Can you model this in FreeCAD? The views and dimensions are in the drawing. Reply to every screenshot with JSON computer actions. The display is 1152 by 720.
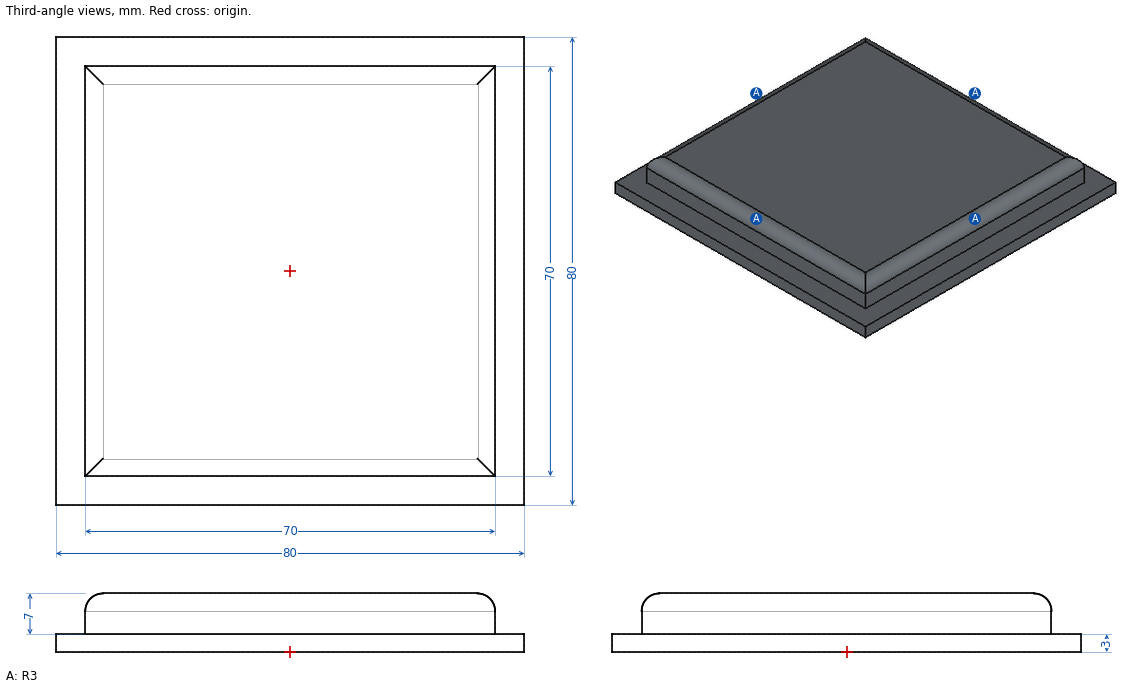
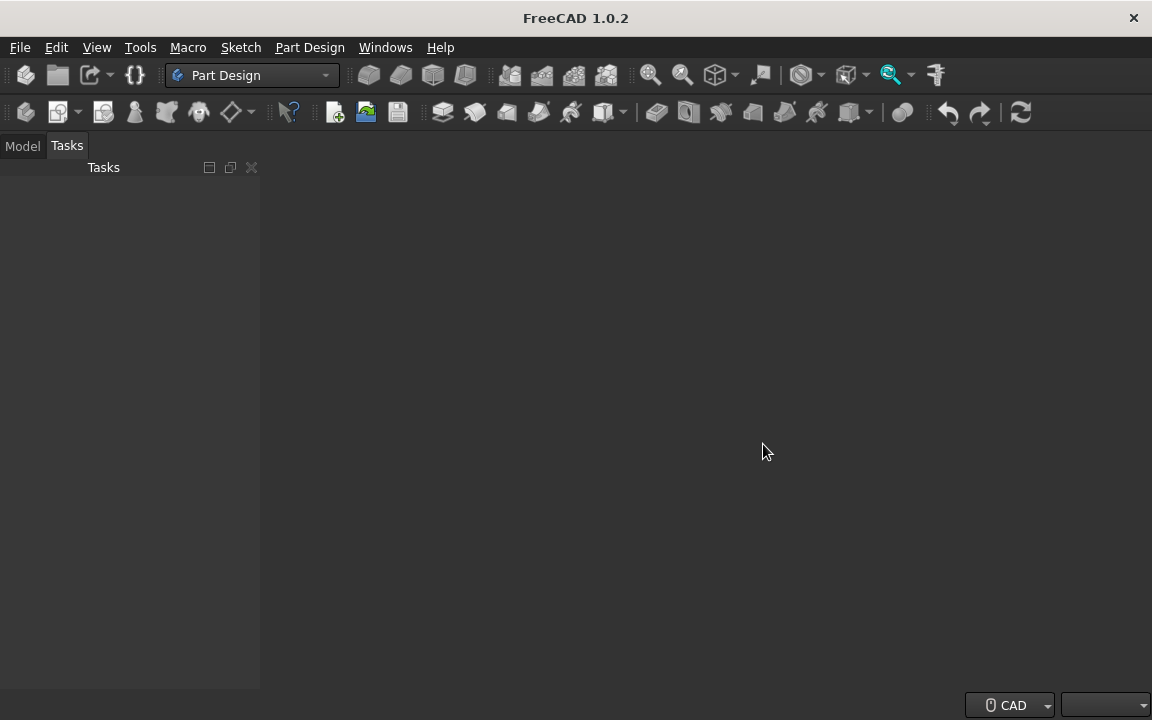
{"action": "left_click", "coordinate": [334, 112]}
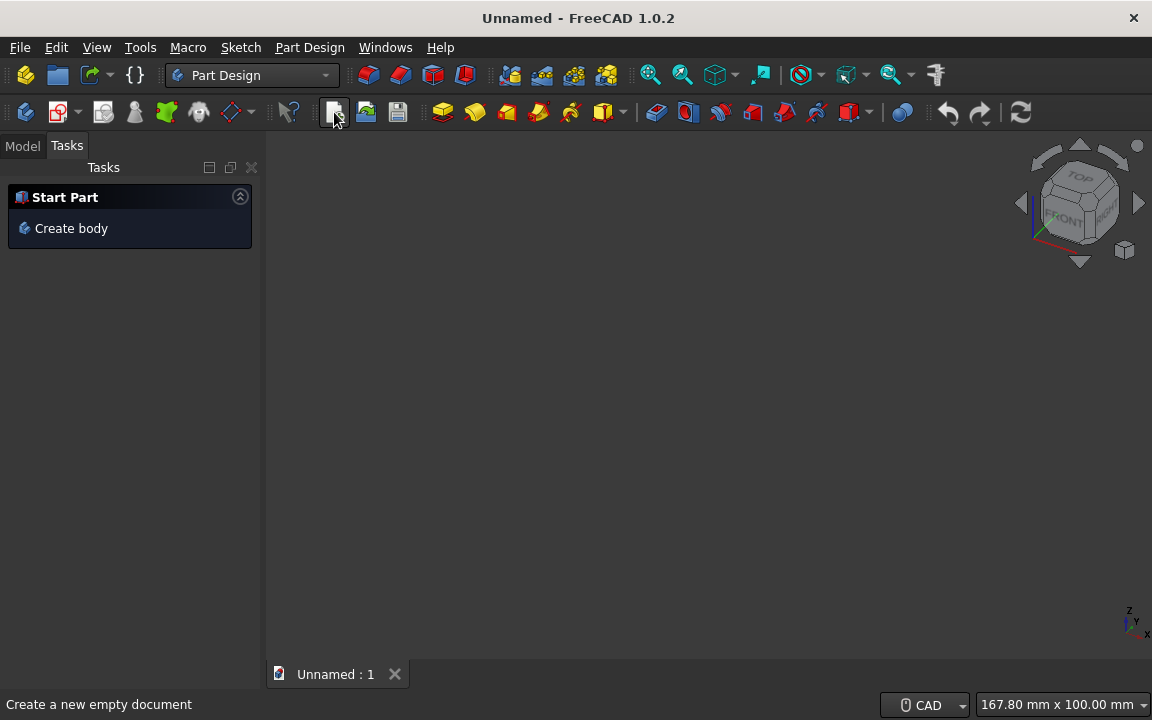
{"action": "left_click", "coordinate": [58, 112]}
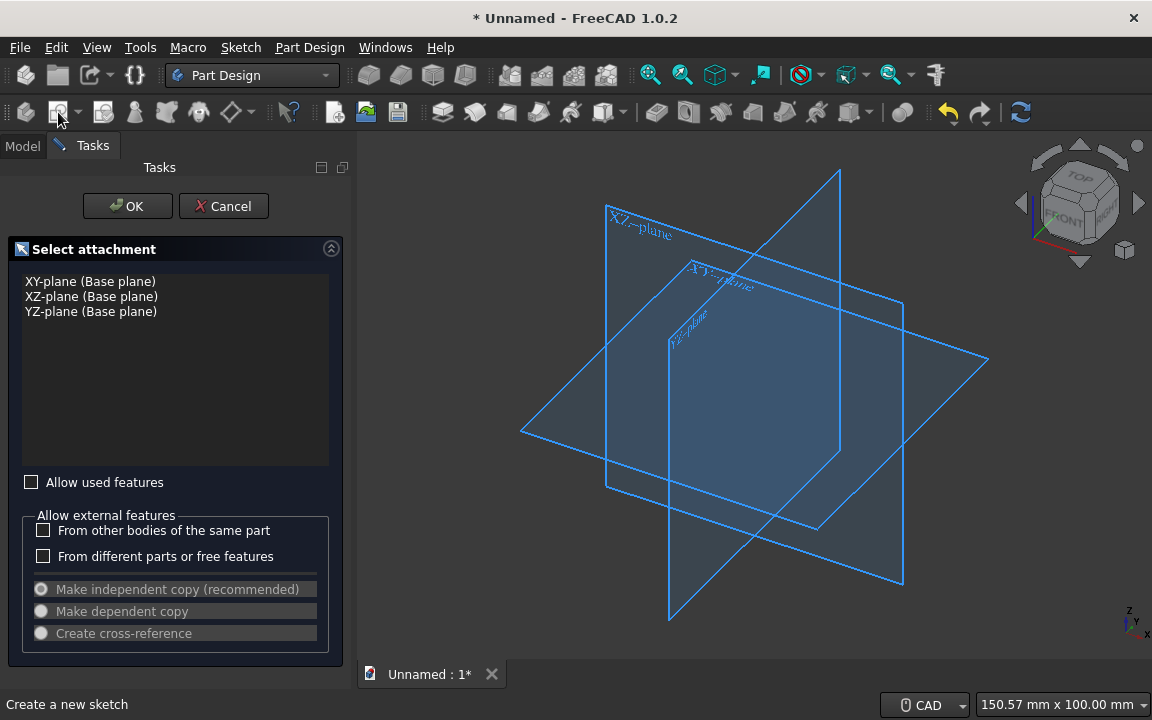
{"action": "left_click", "coordinate": [82, 282]}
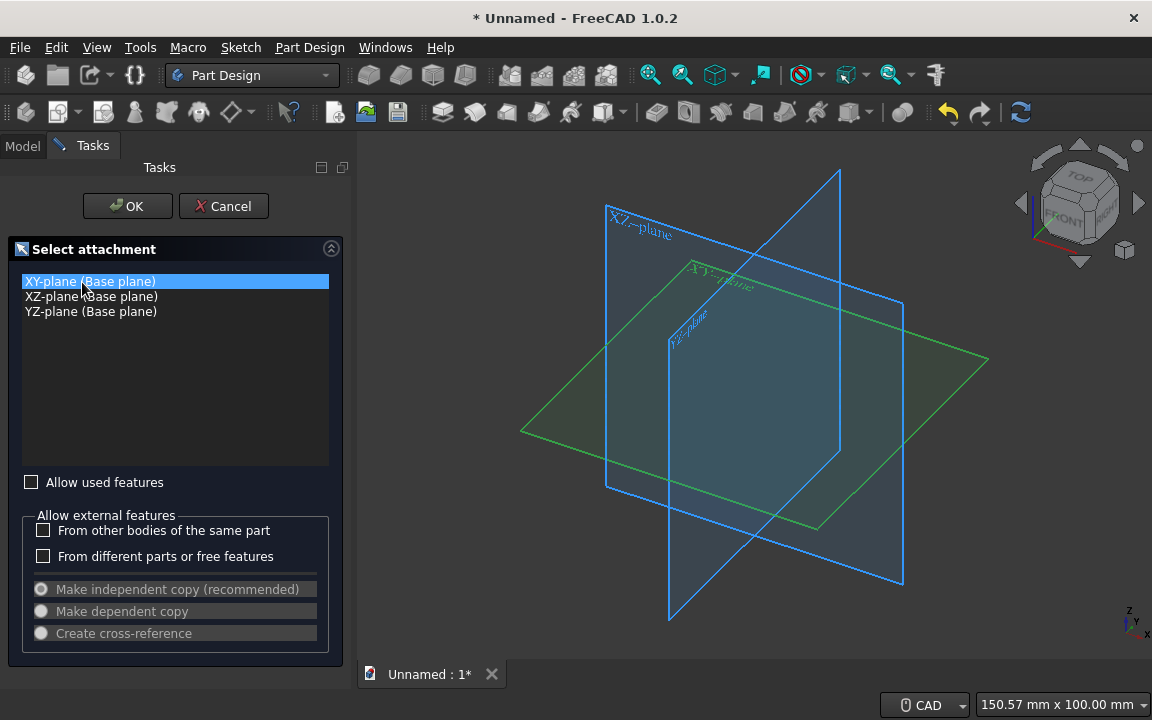
{"action": "left_click", "coordinate": [128, 206]}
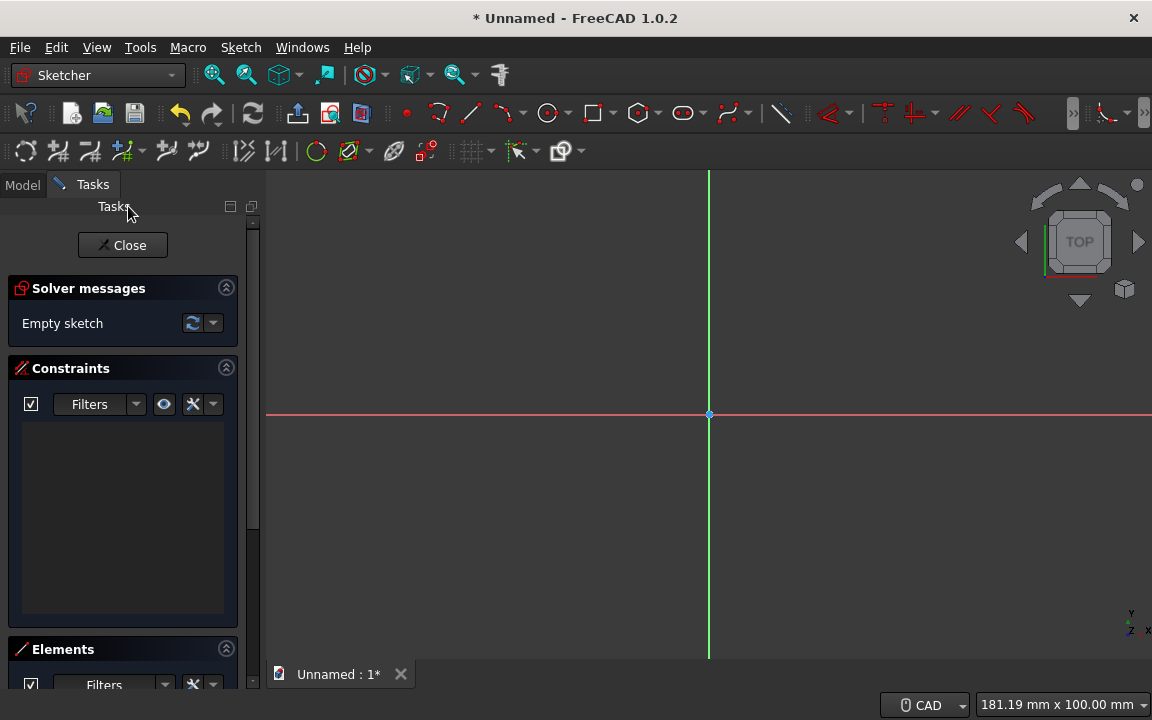
{"action": "scroll", "coordinate": [331, 415], "scroll_direction": "down", "scroll_amount": 1}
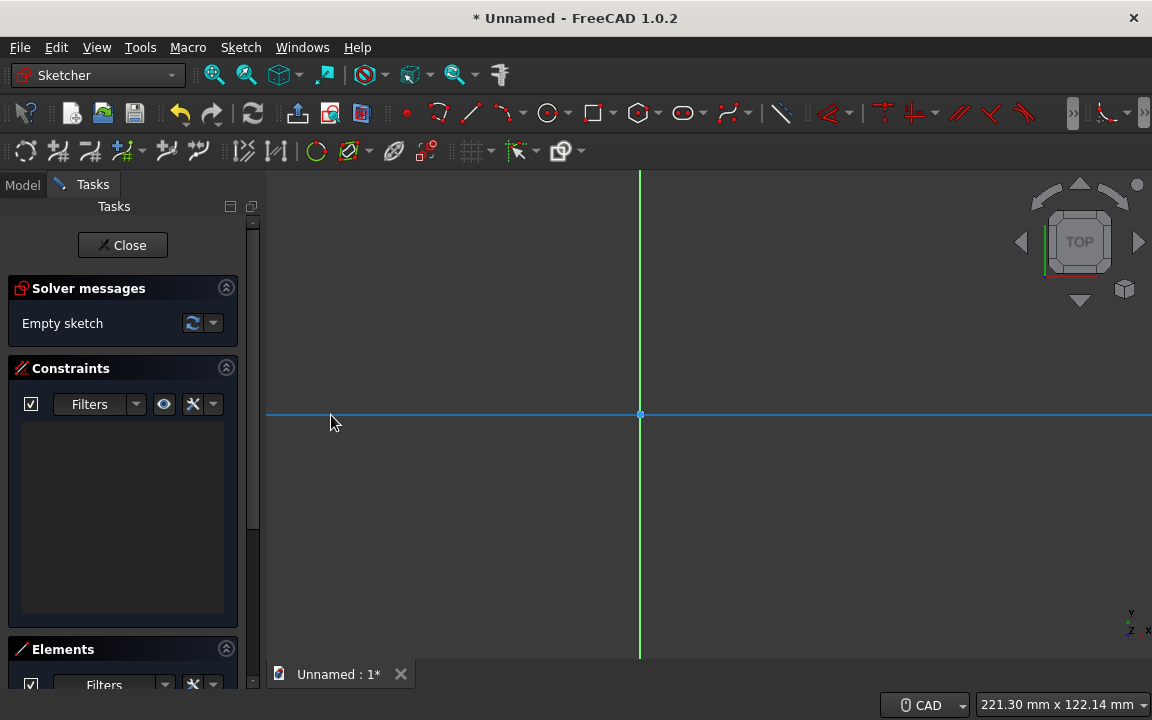
{"action": "left_click", "coordinate": [616, 114]}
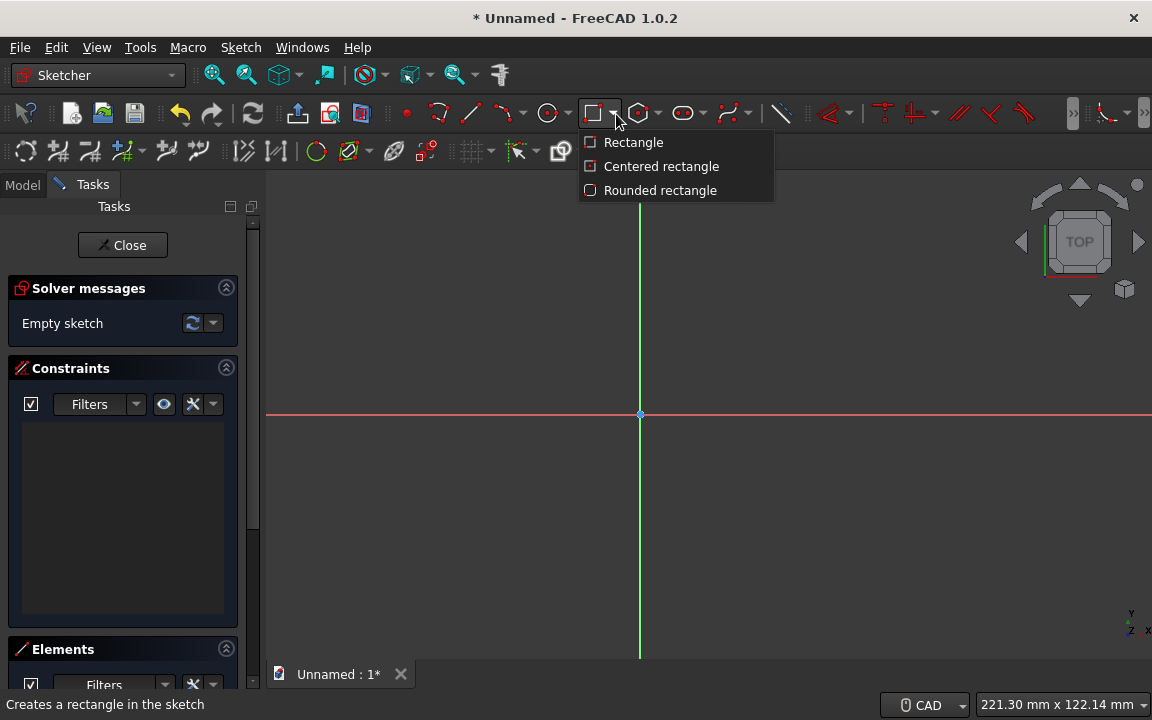
{"action": "left_click", "coordinate": [676, 166]}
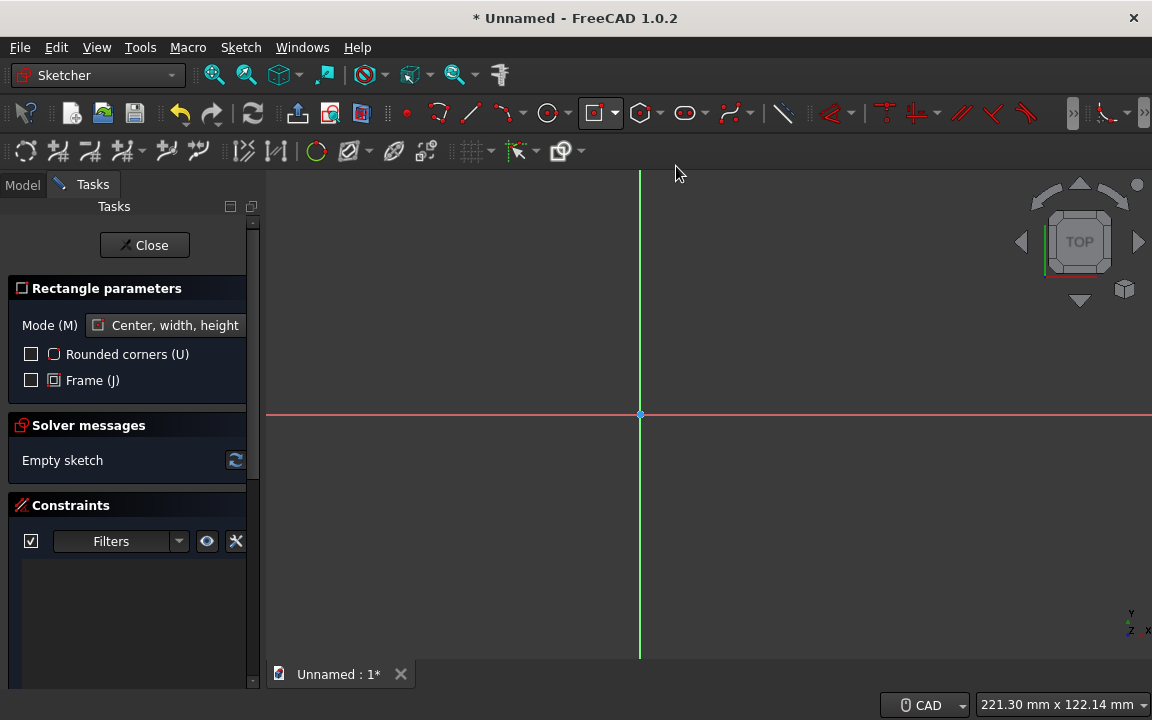
{"action": "left_click", "coordinate": [640, 415]}
{"action": "left_click", "coordinate": [801, 255]}
{"action": "key", "text": "Escape"}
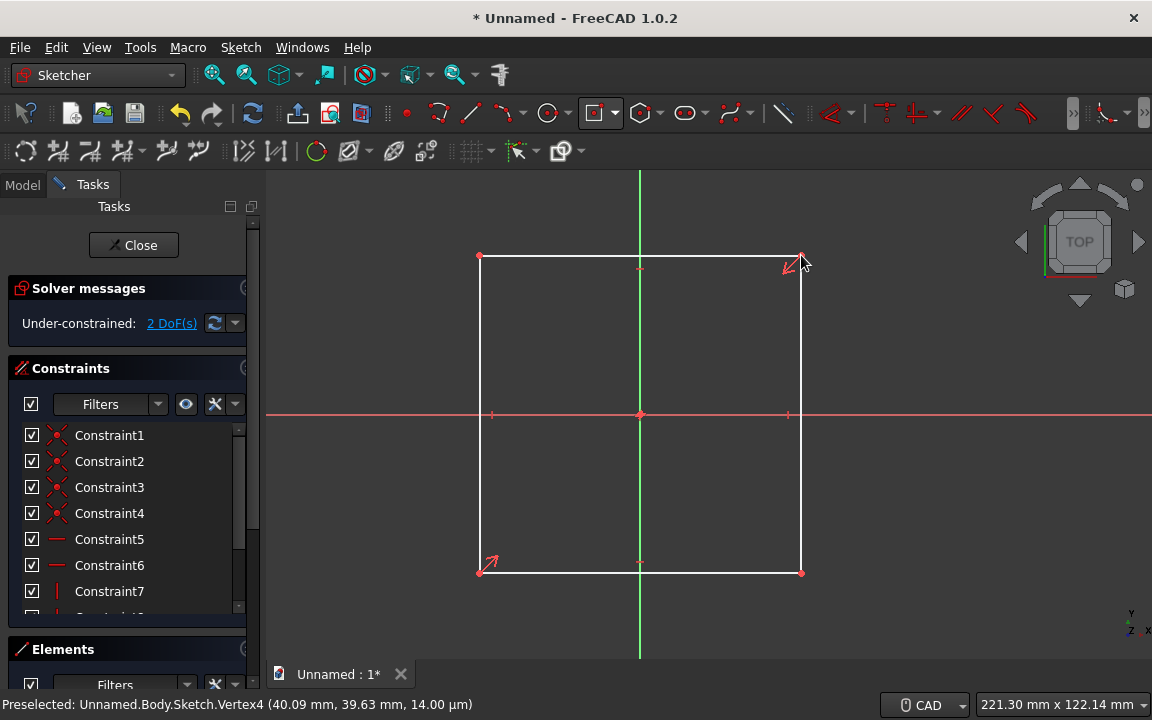
{"action": "left_click", "coordinate": [830, 114]}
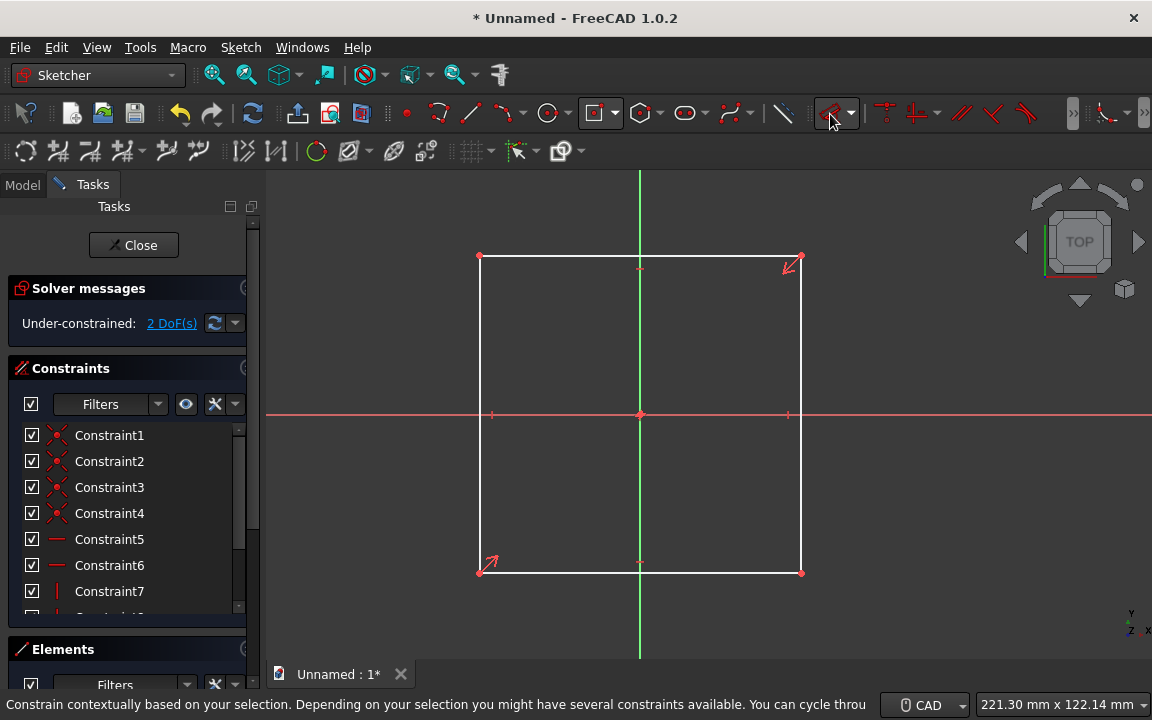
{"action": "left_click", "coordinate": [576, 573]}
{"action": "left_click", "coordinate": [567, 607]}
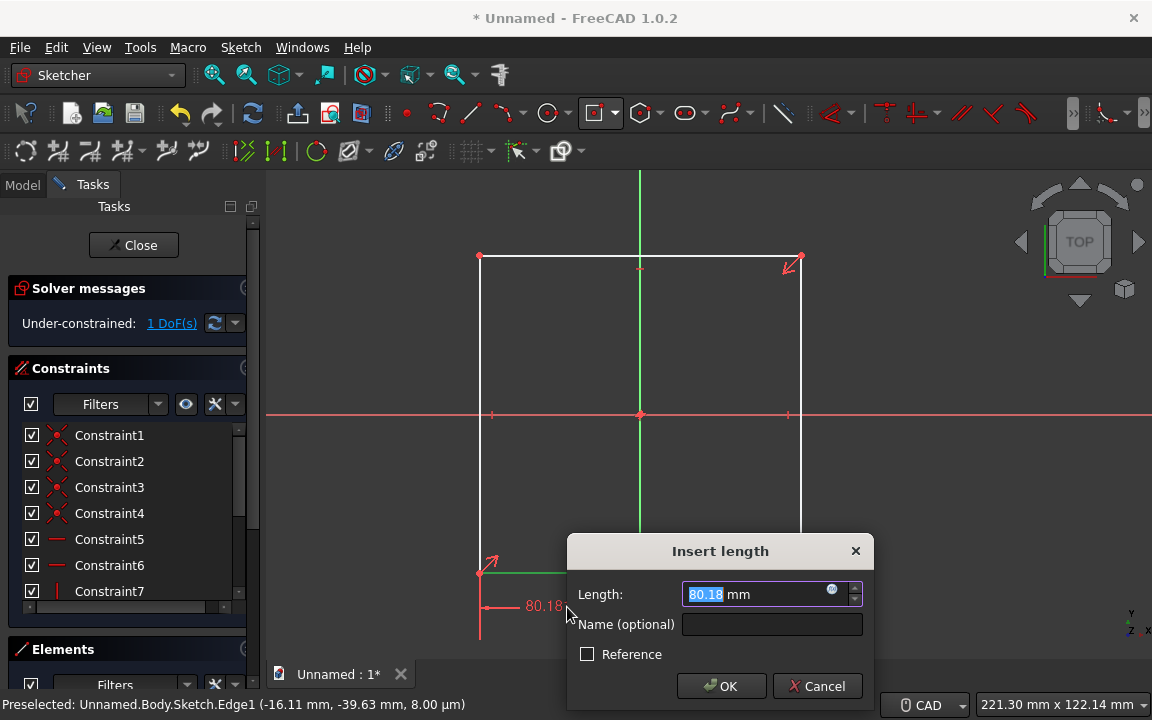
{"action": "type", "text": "80"}
{"action": "key", "text": "Return"}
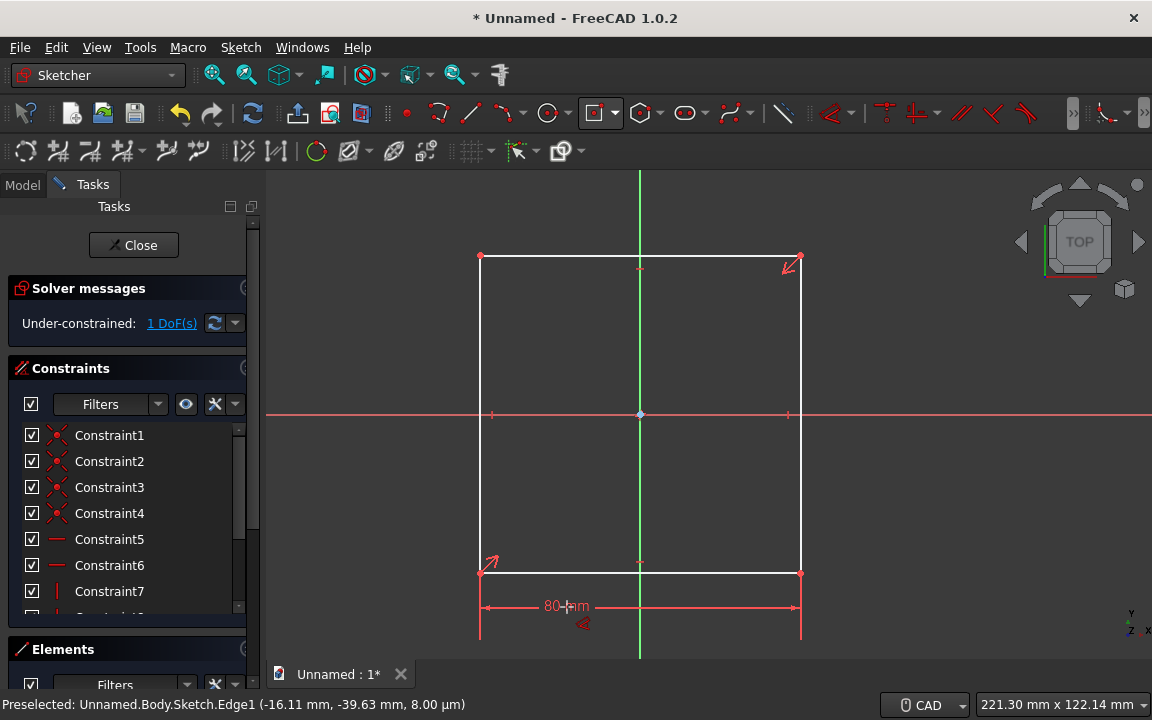
{"action": "left_click", "coordinate": [801, 478]}
{"action": "left_click", "coordinate": [835, 342]}